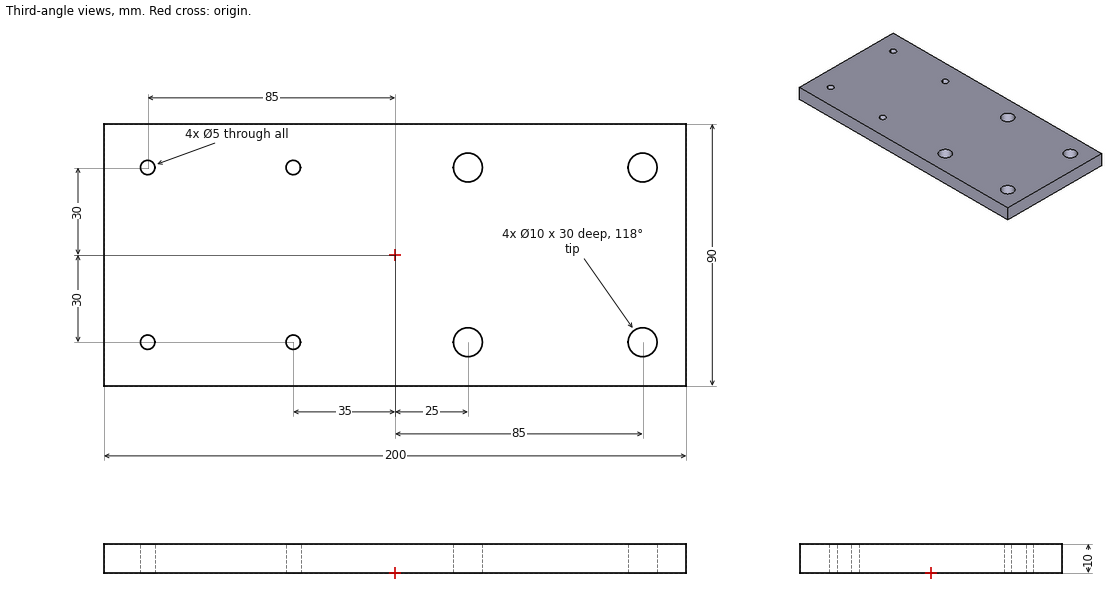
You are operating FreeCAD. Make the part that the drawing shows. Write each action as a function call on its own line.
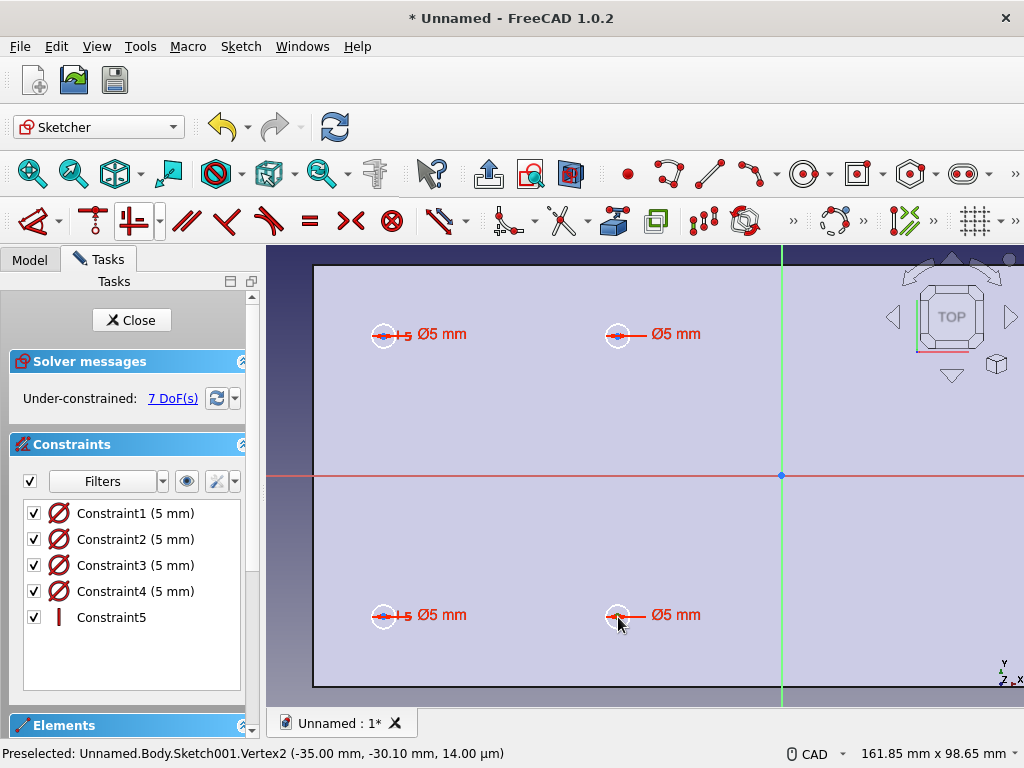
click(384, 617)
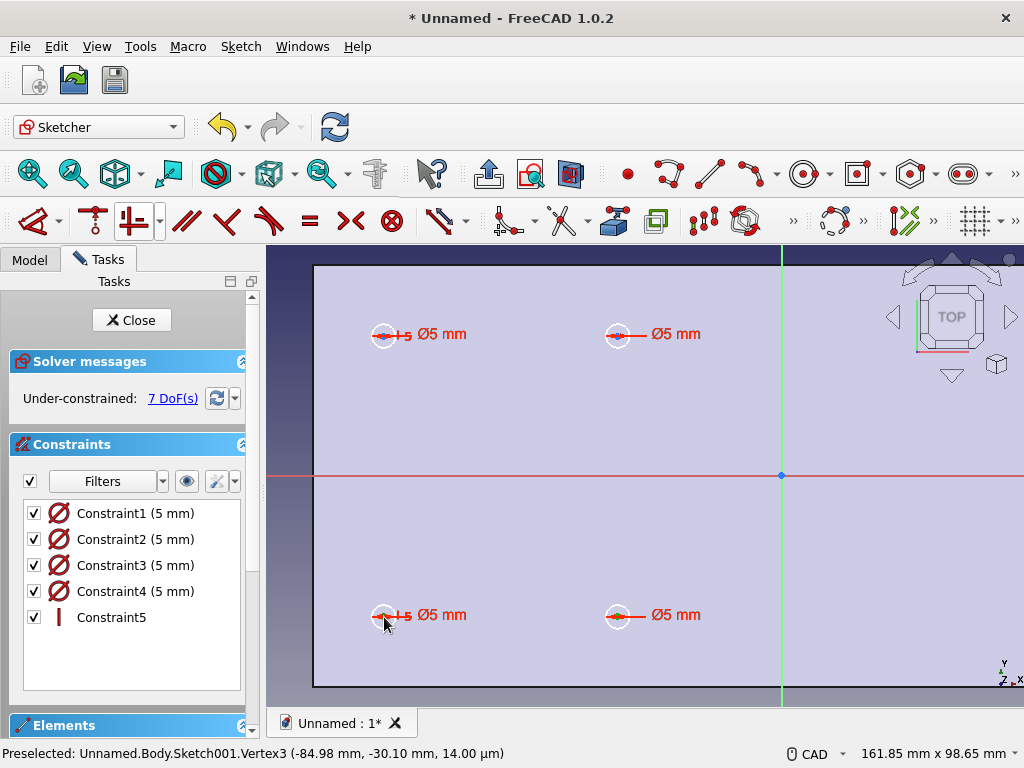
key(h)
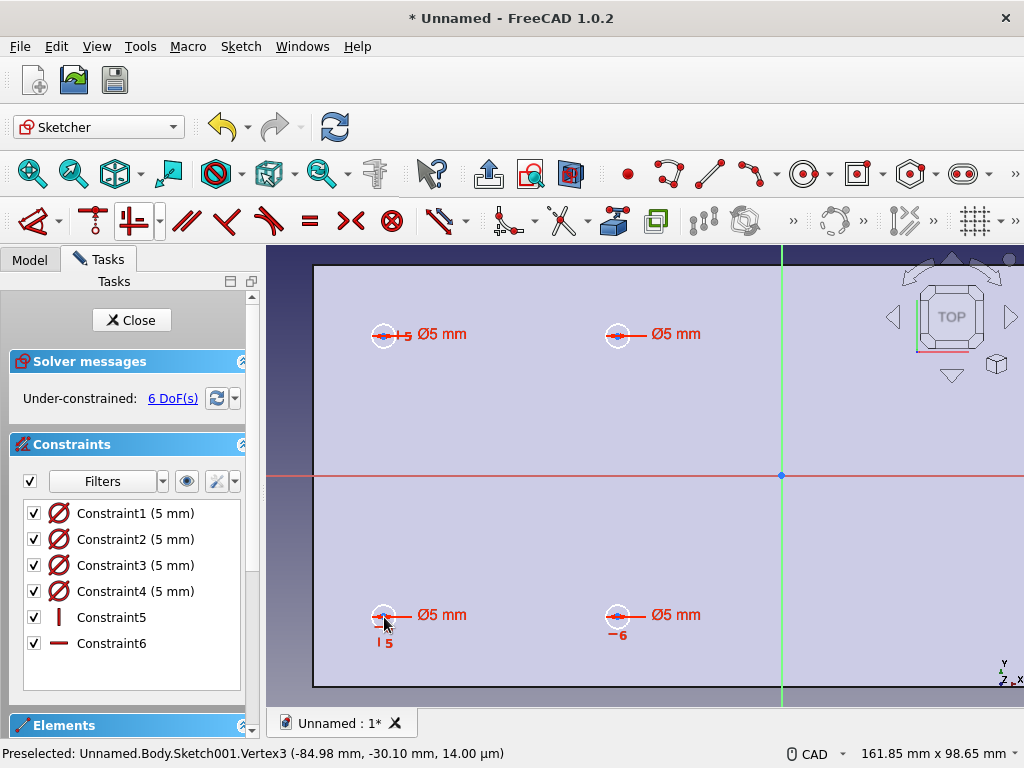
click(618, 617)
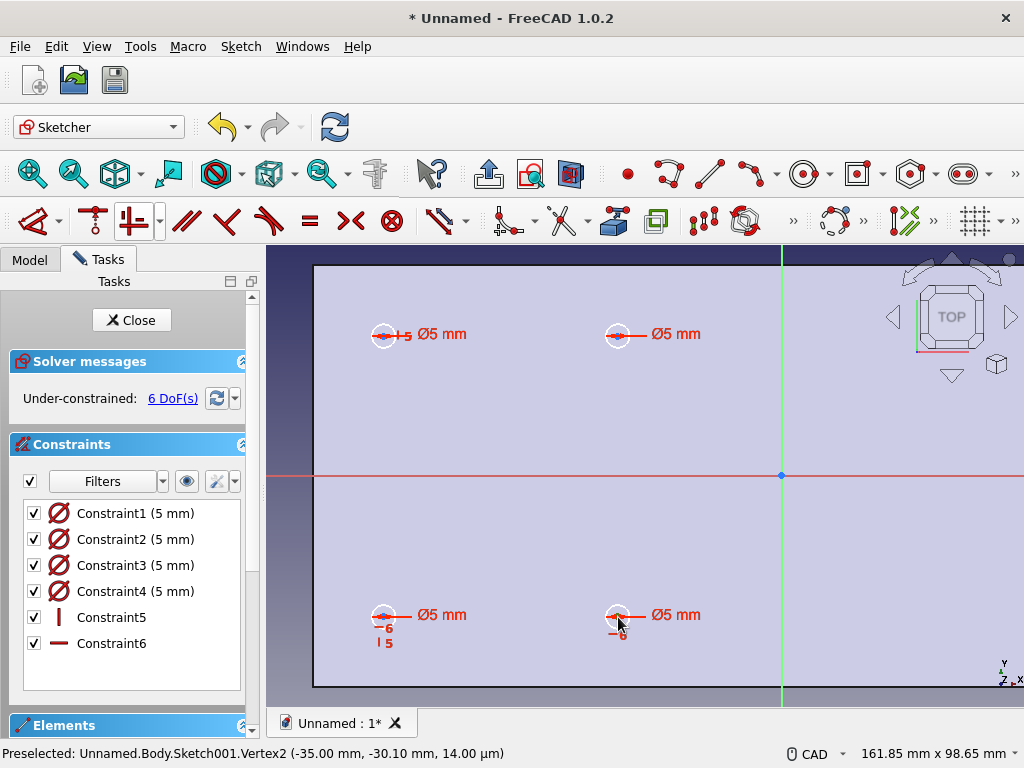
click(618, 336)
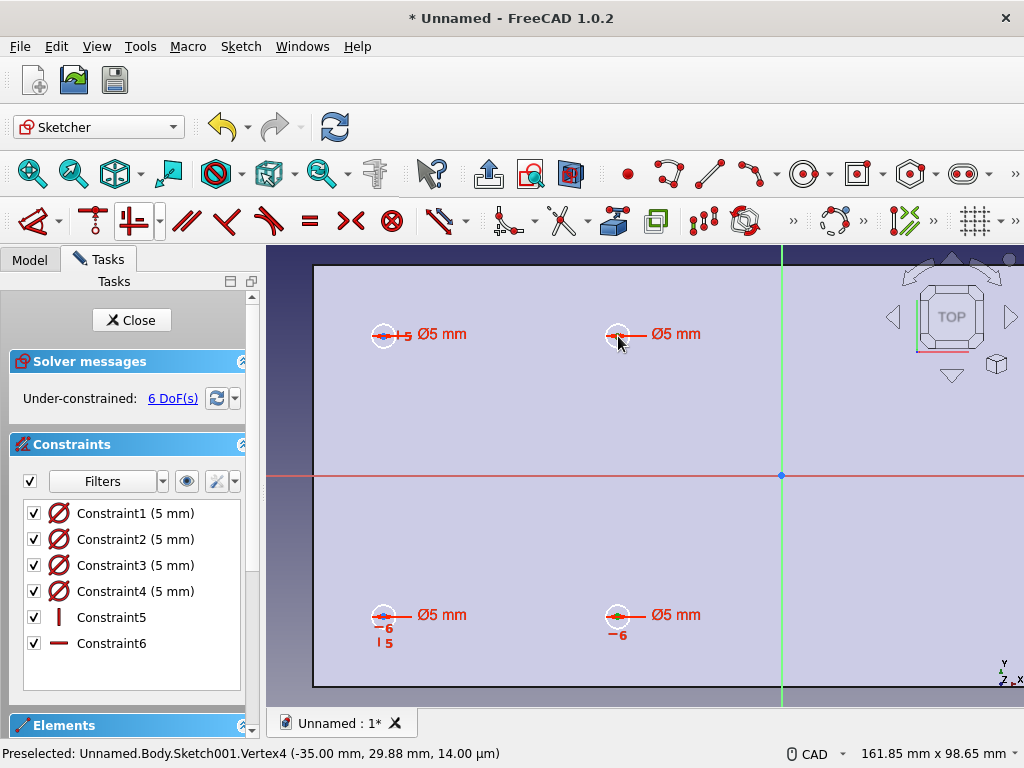
key(v)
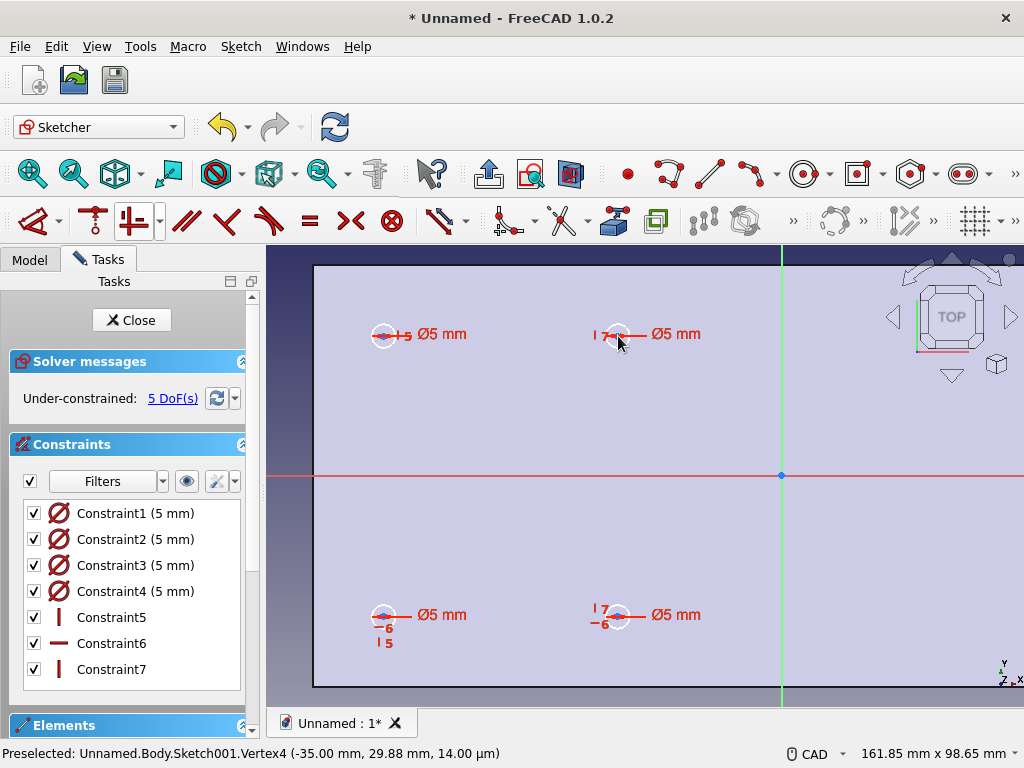
click(384, 336)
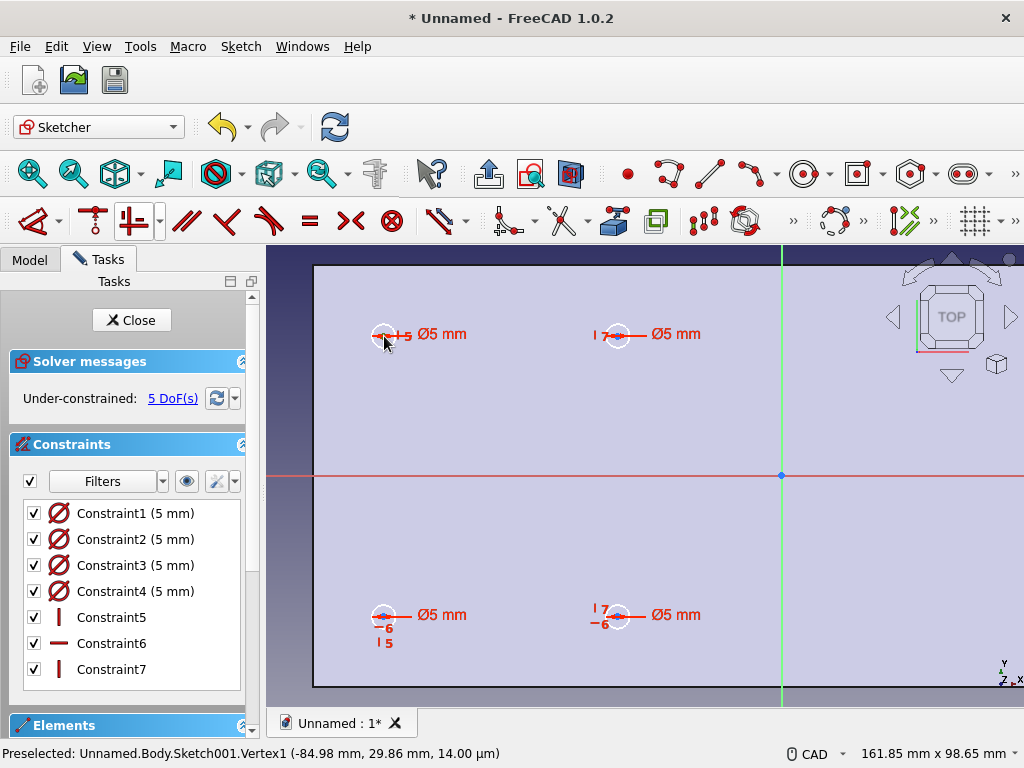
click(618, 336)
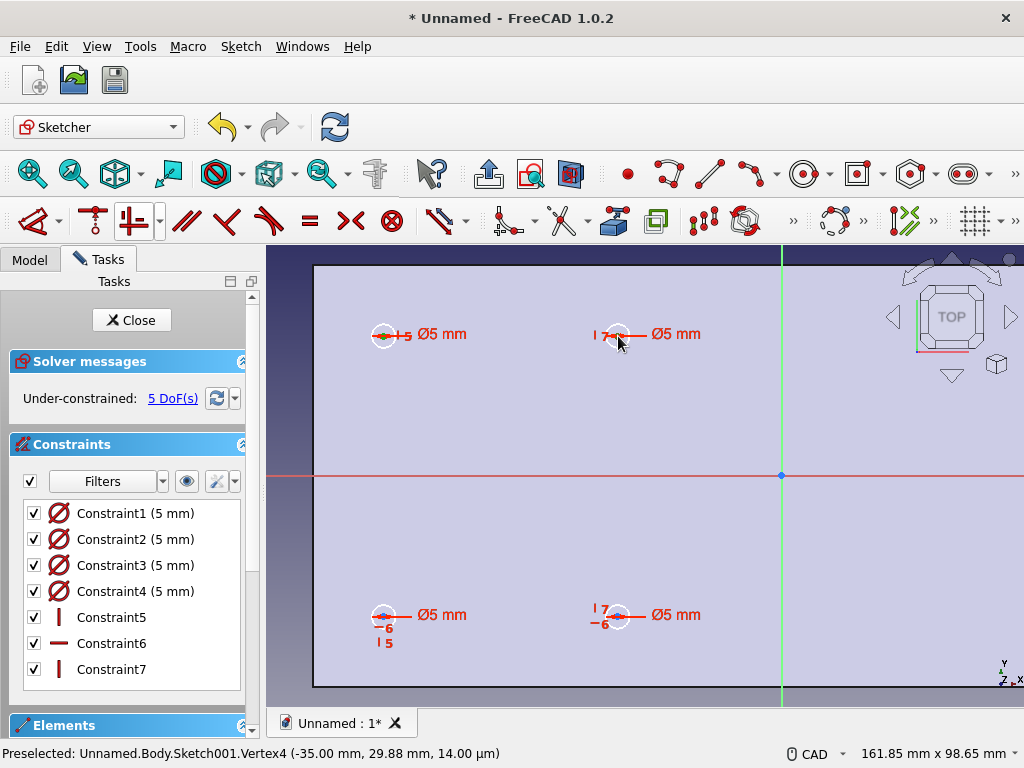
key(h)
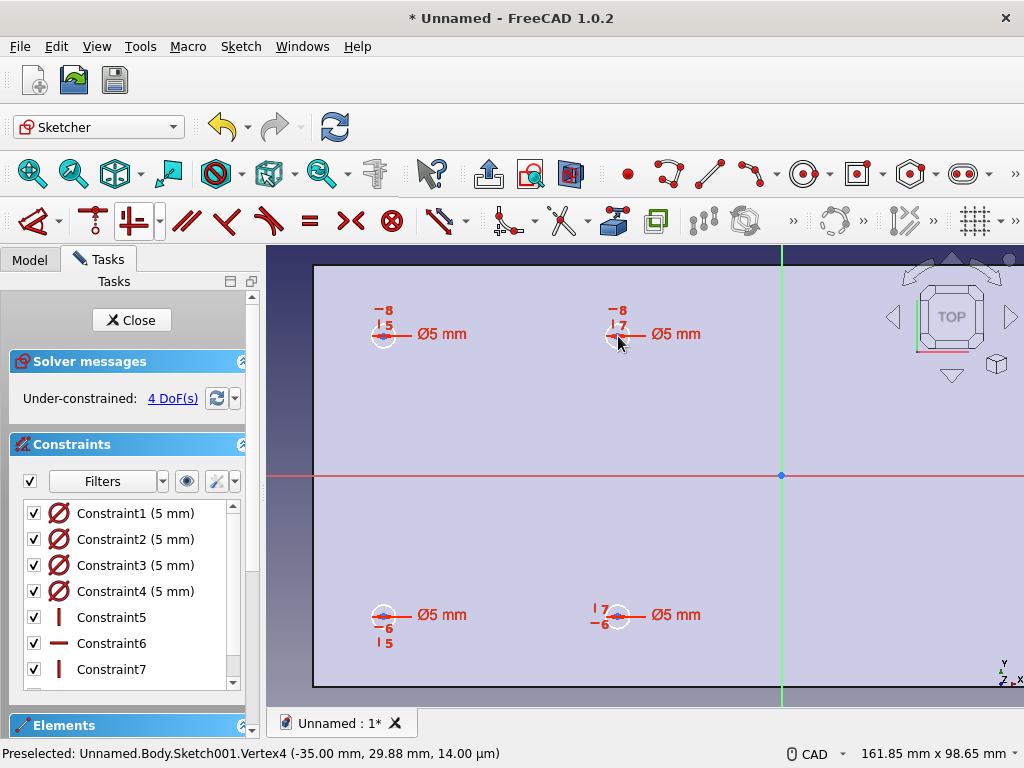
click(32, 222)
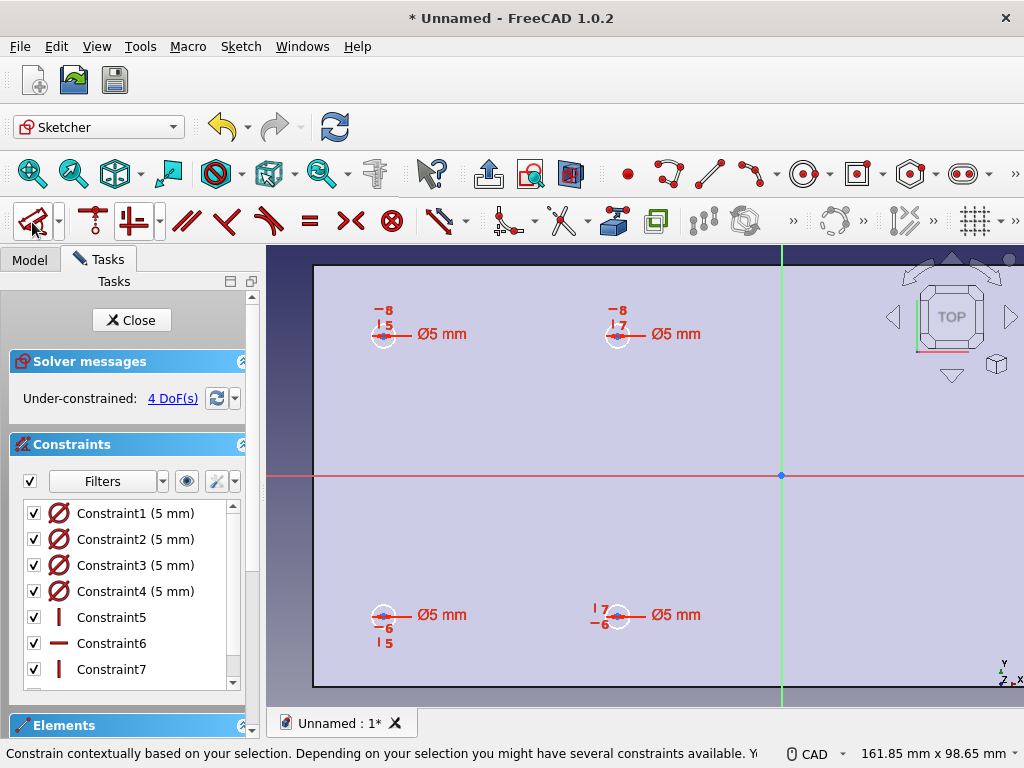
click(384, 336)
click(583, 302)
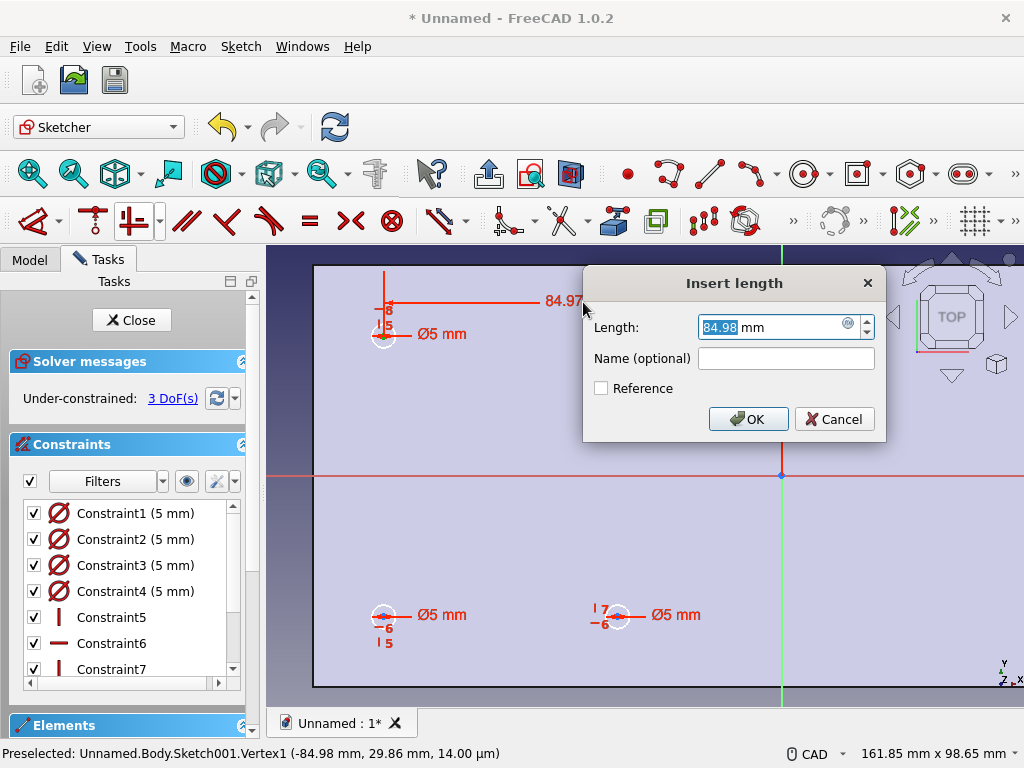
text(85)
key(Return)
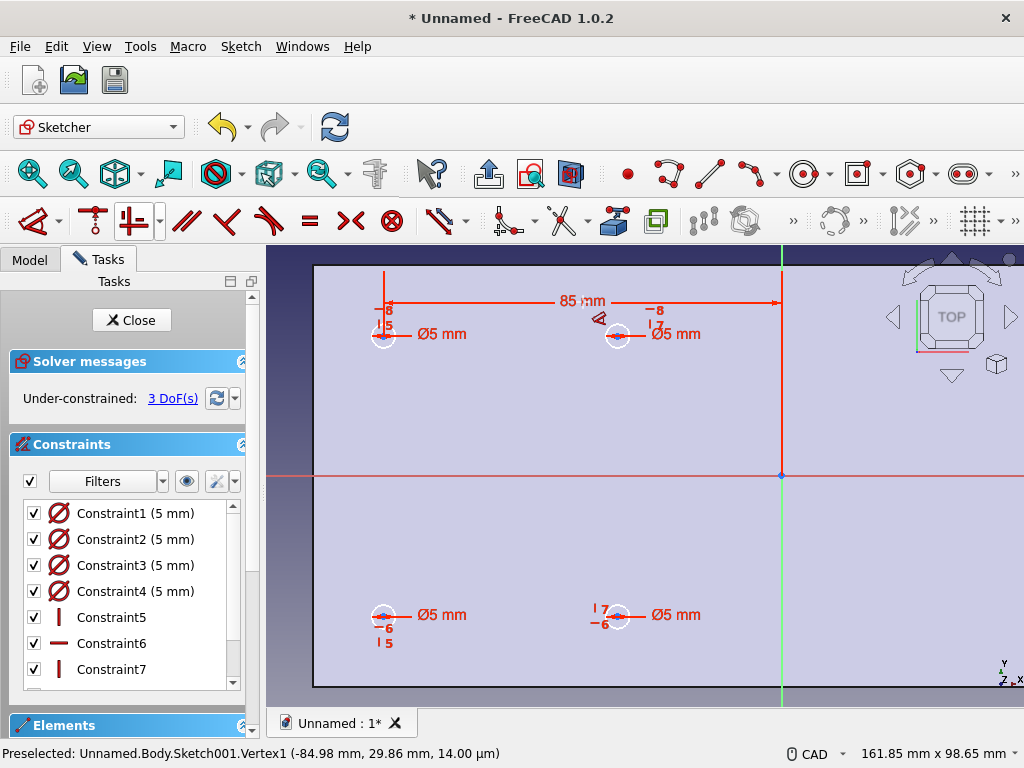
click(384, 336)
click(816, 406)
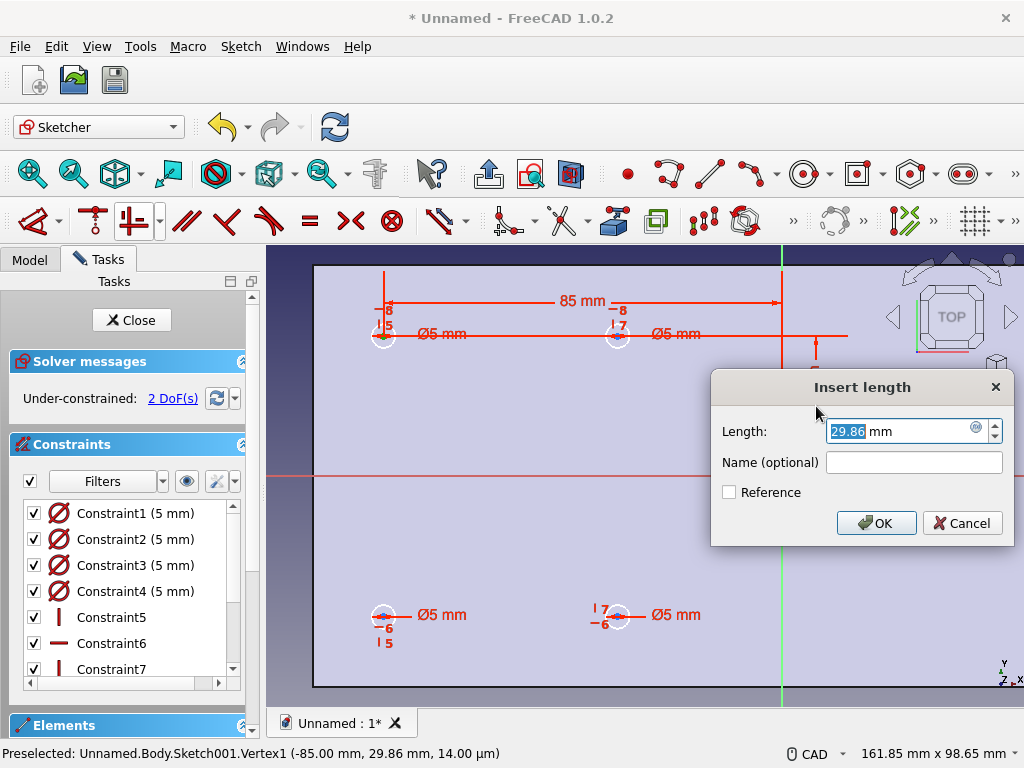
text(30)
key(Return)